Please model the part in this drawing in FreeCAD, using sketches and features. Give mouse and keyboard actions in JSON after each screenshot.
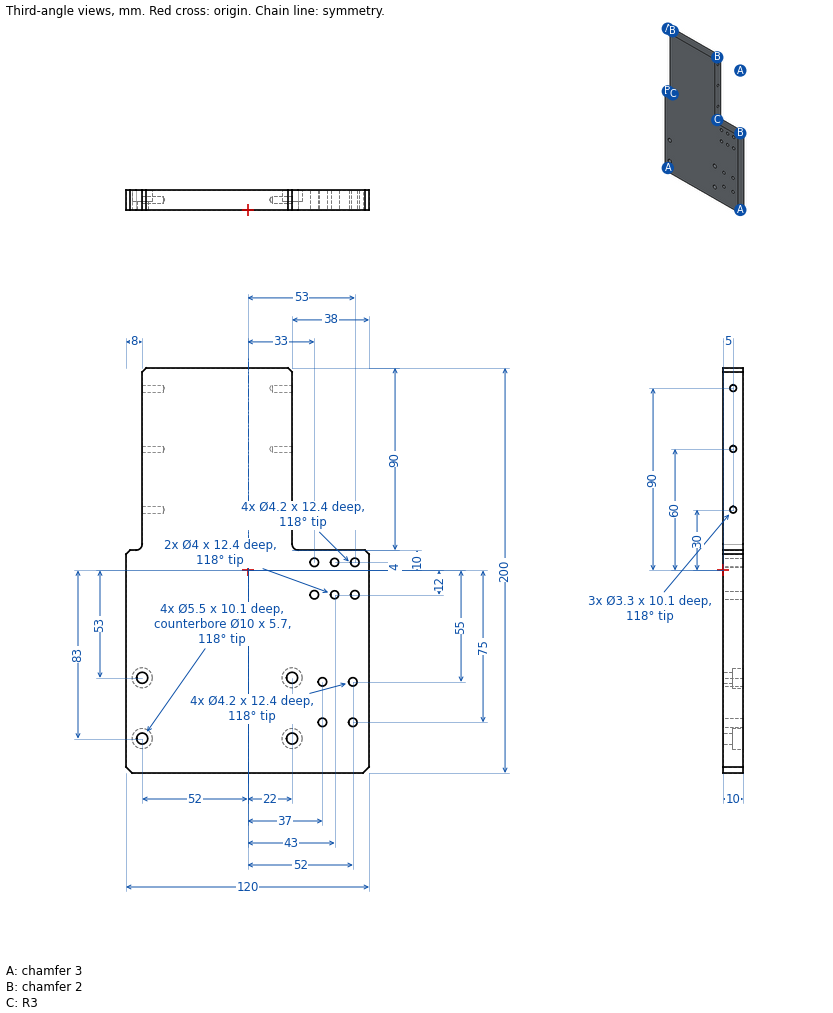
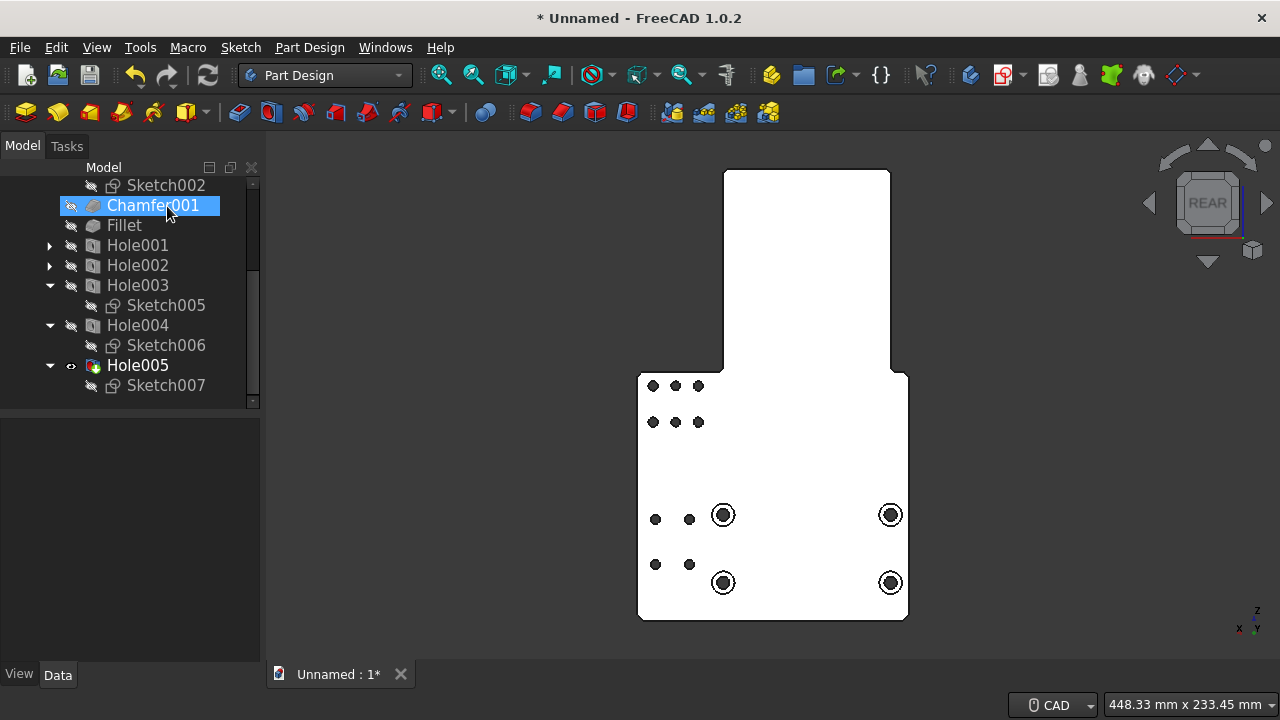
{"action": "key", "text": "0"}